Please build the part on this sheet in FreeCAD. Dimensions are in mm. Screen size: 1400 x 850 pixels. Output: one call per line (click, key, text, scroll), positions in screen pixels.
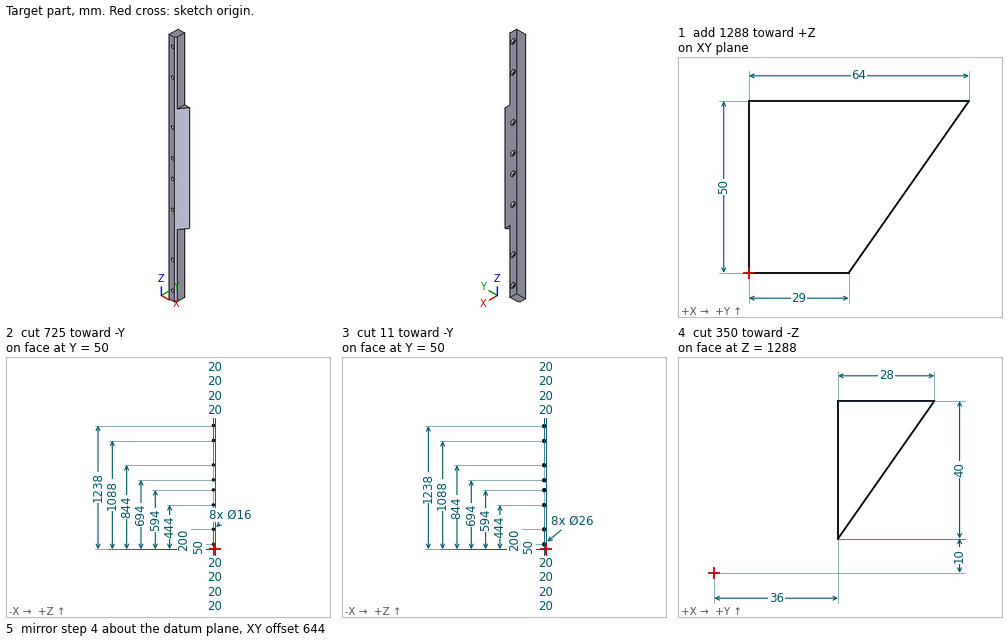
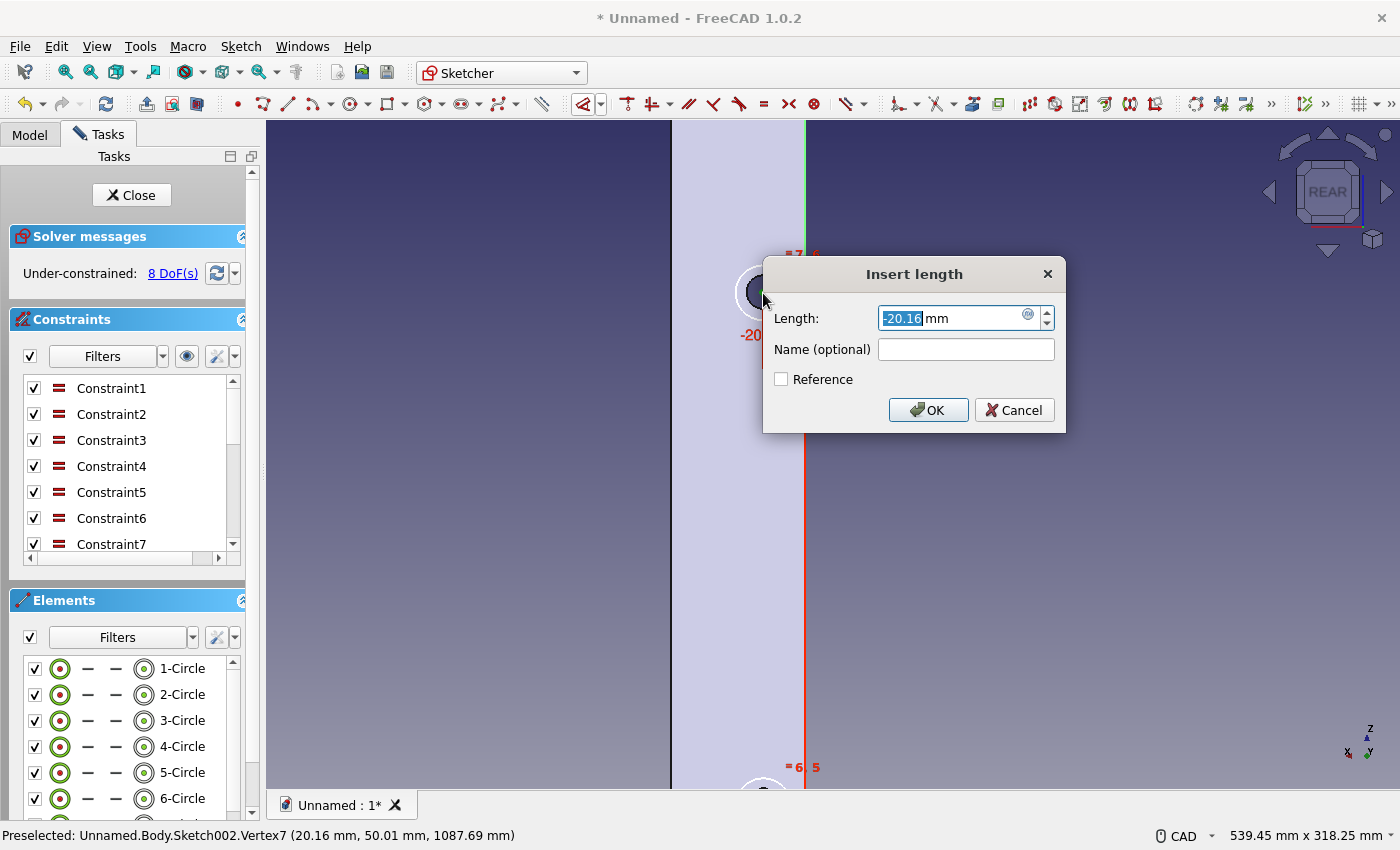
text(-20)
key(Return)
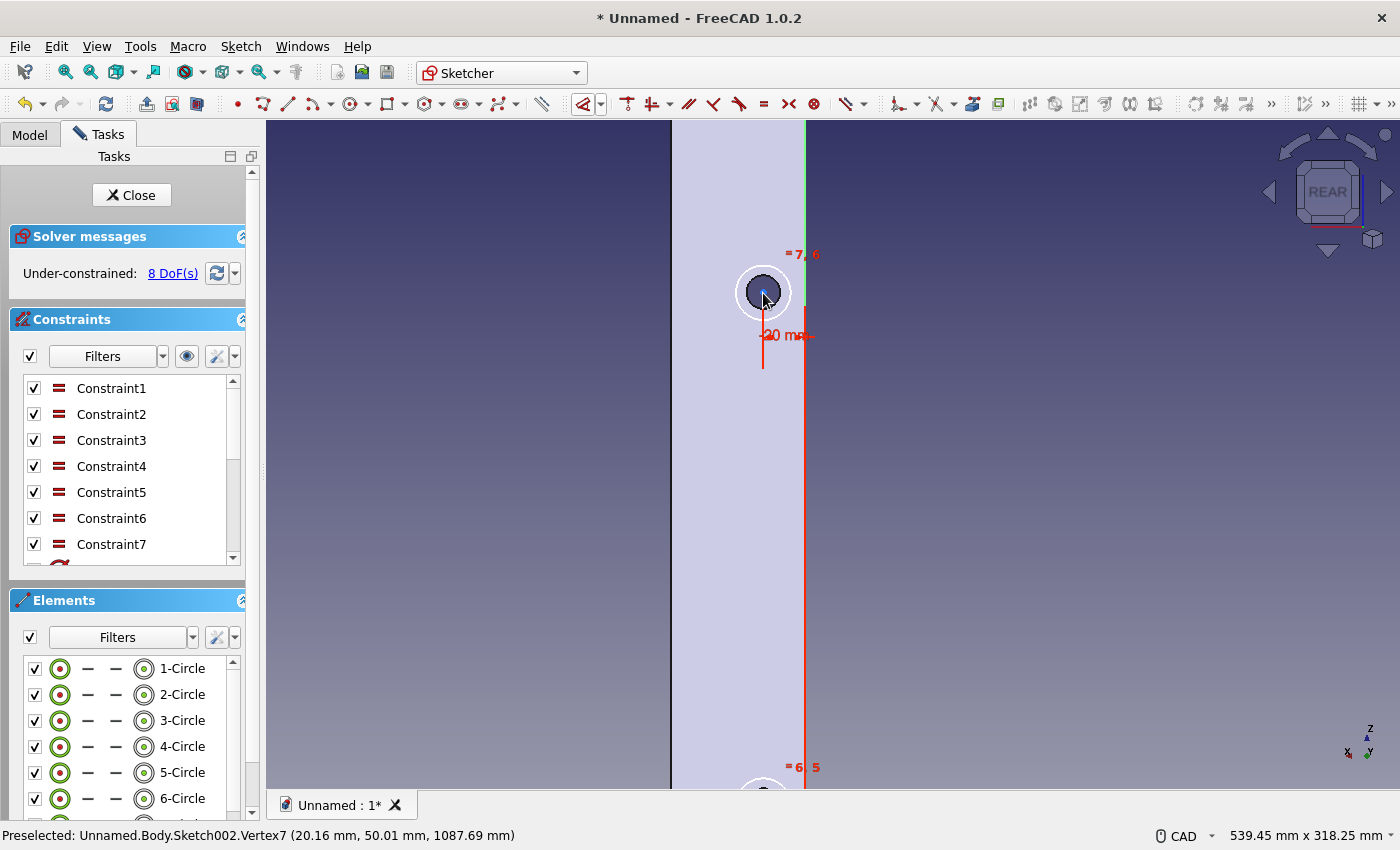
scroll(763, 294, down, 9)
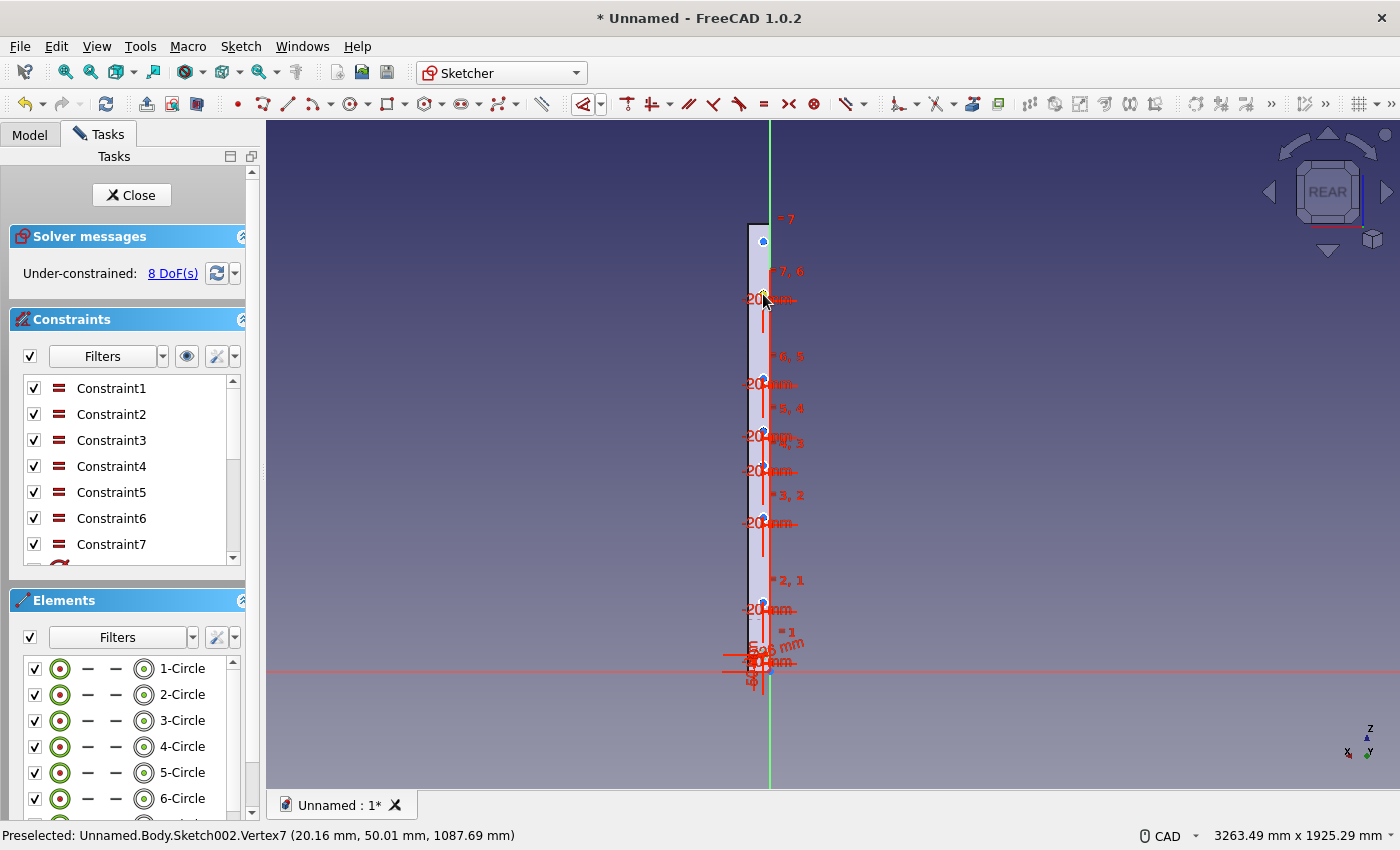
scroll(763, 242, up, 9)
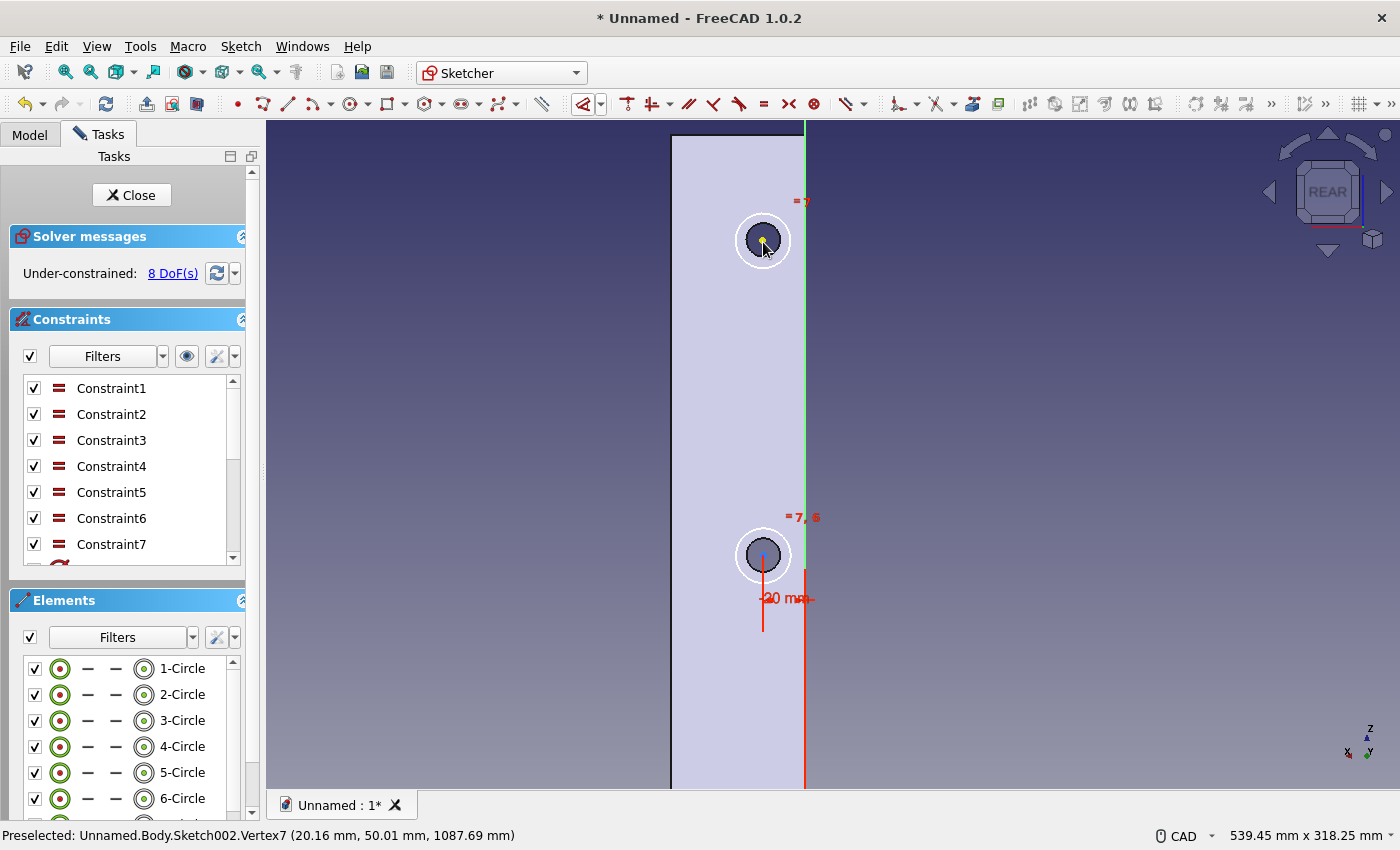
click(763, 241)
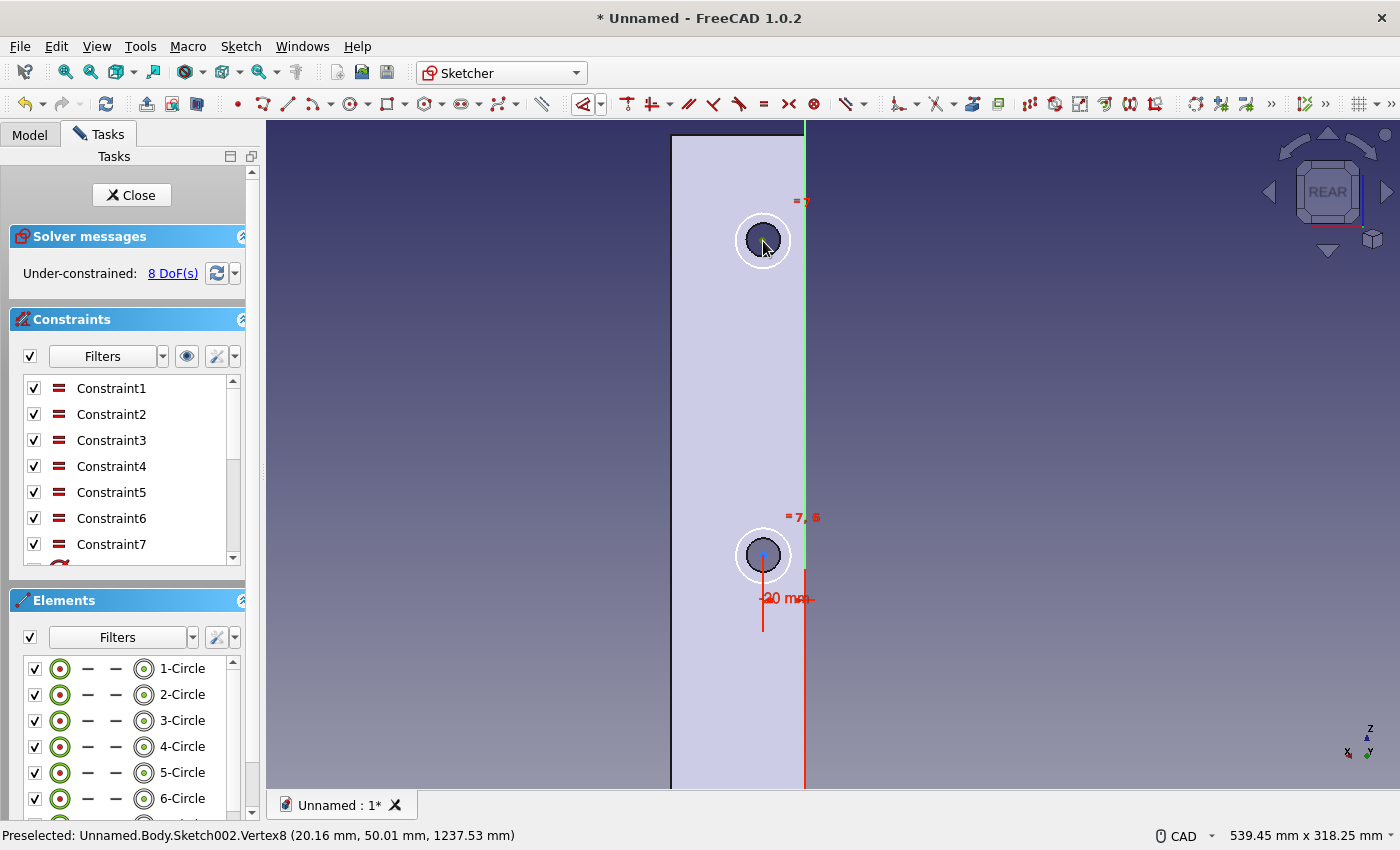
key(l)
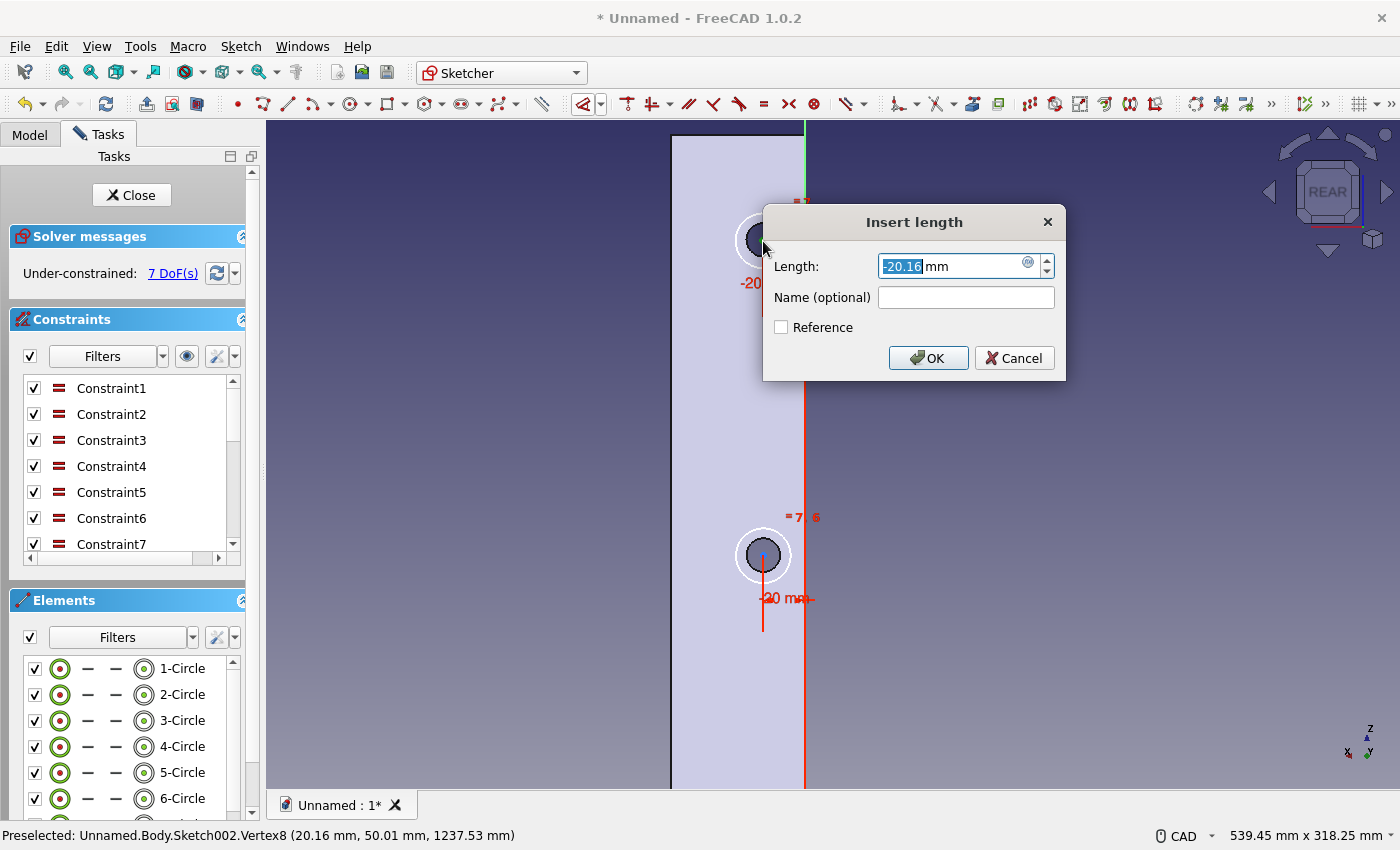
text(-20)
key(Return)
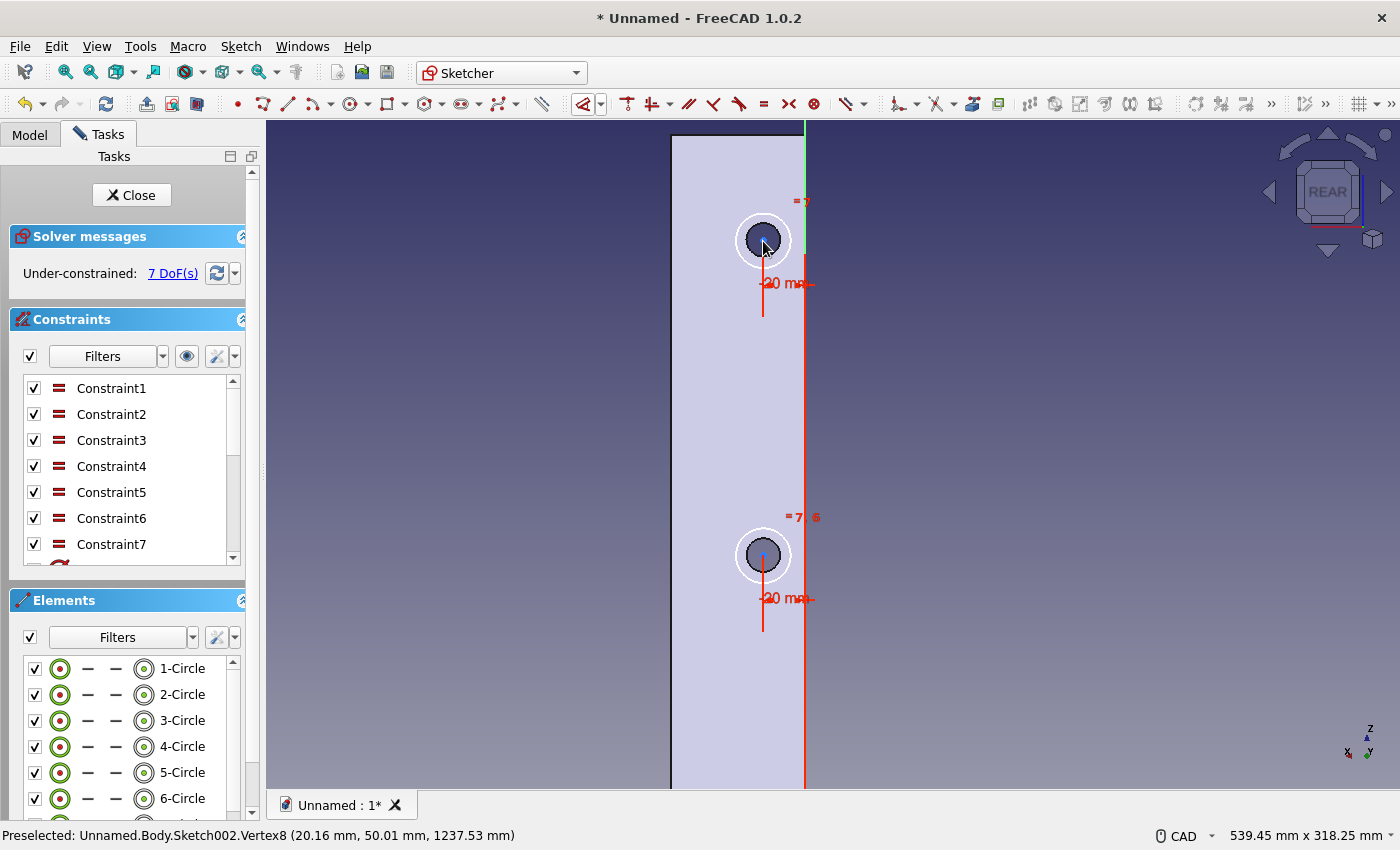
scroll(763, 242, down, 9)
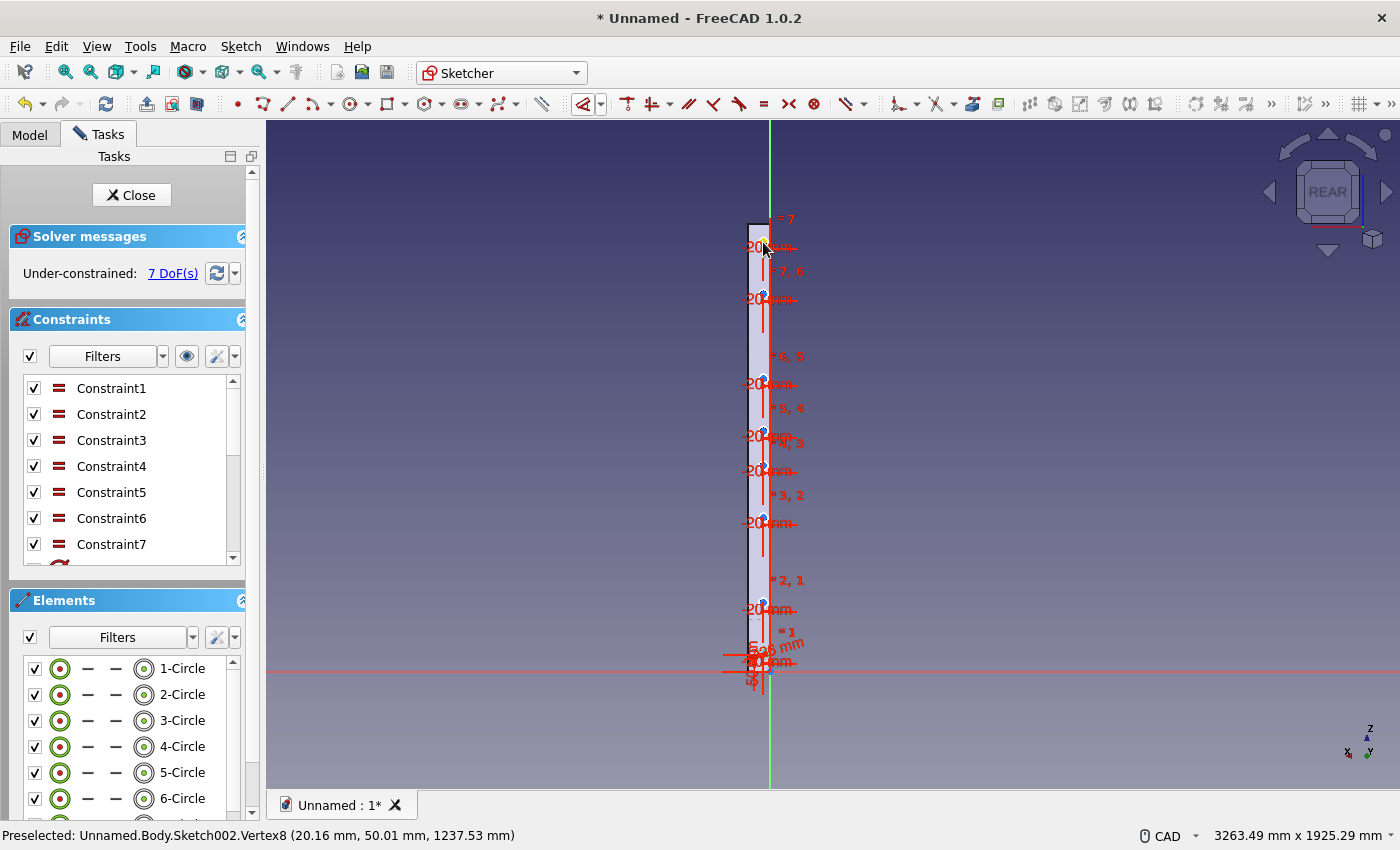
click(763, 603)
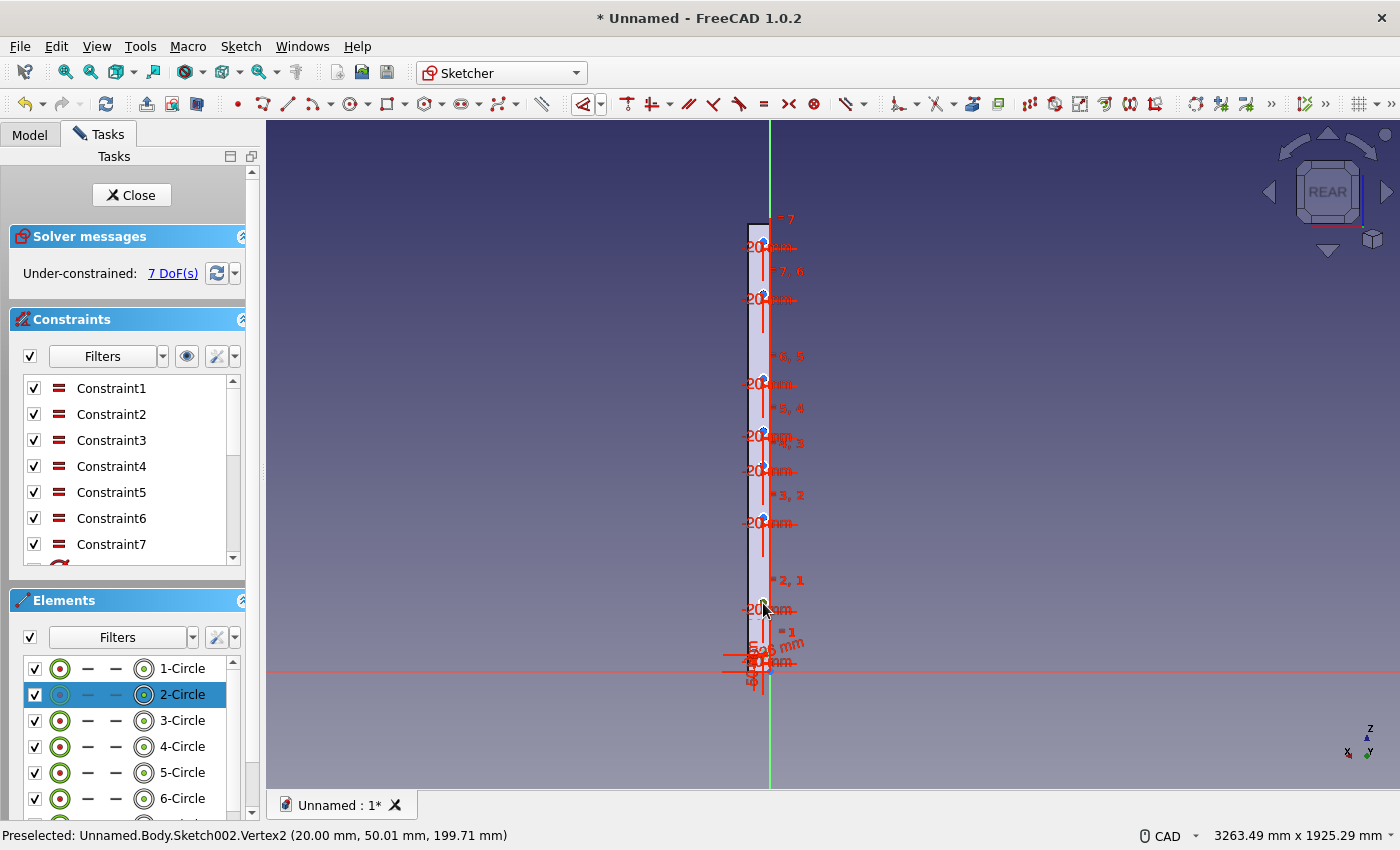
key(i)